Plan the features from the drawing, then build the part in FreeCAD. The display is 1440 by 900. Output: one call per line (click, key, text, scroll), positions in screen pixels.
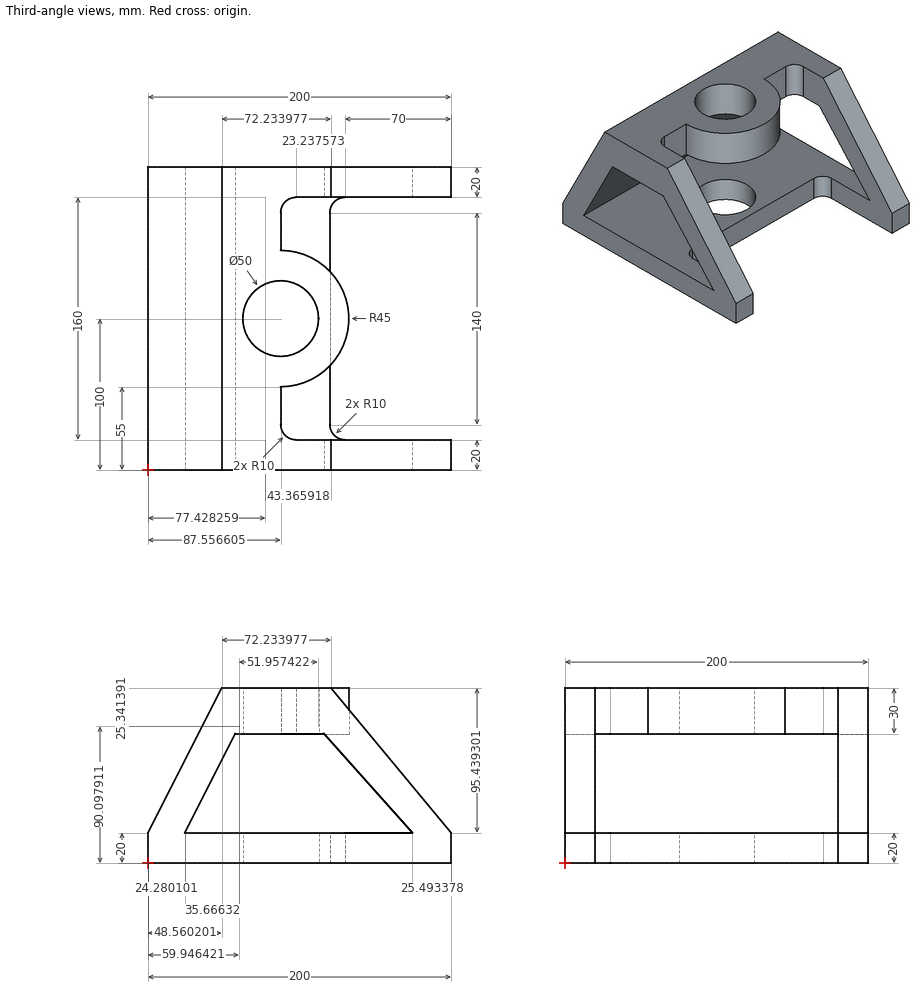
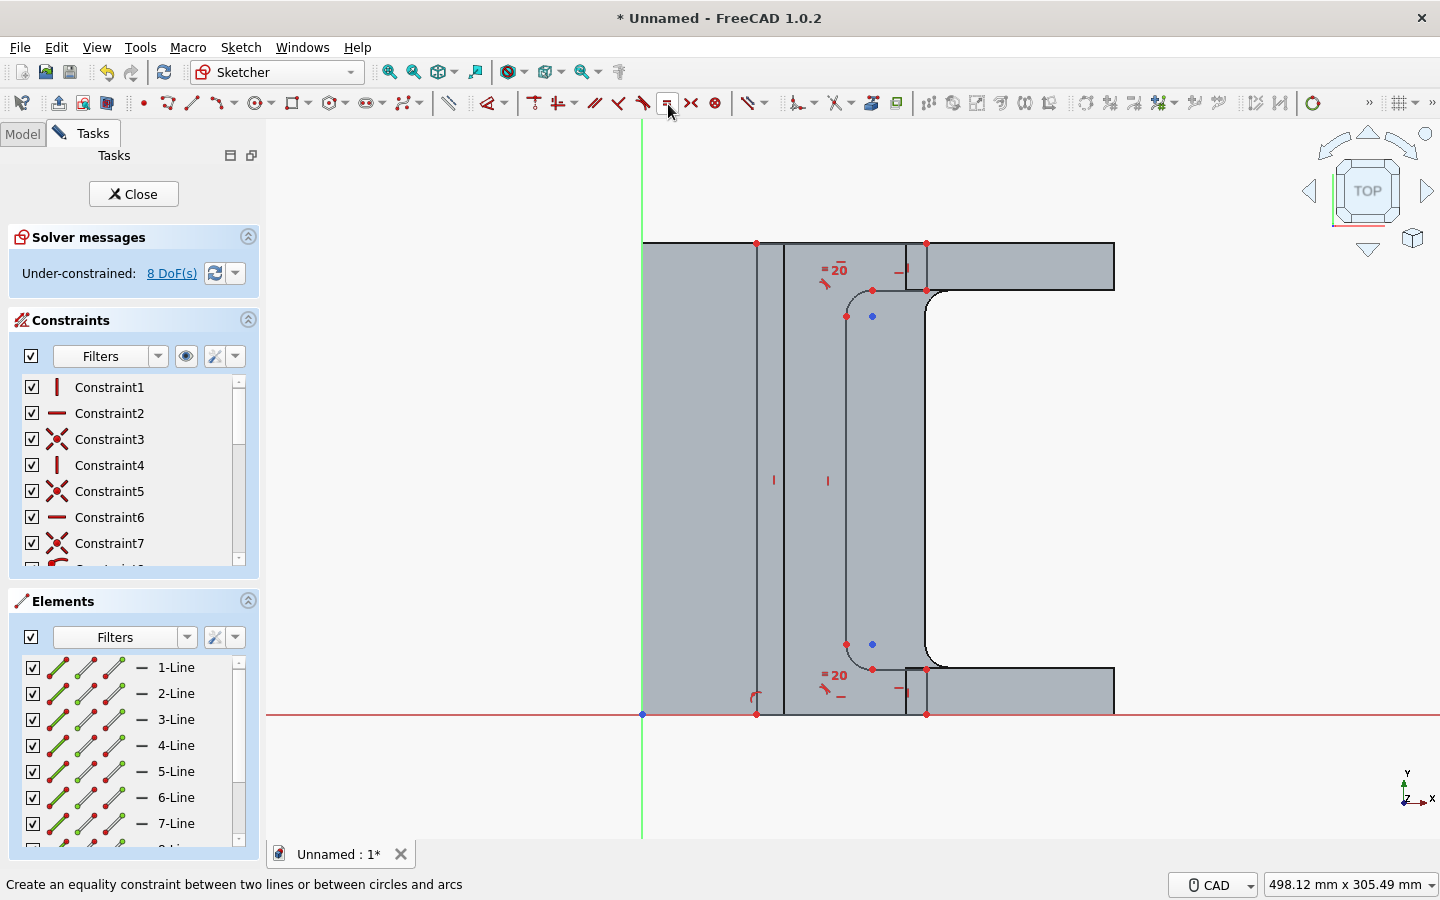
click(488, 104)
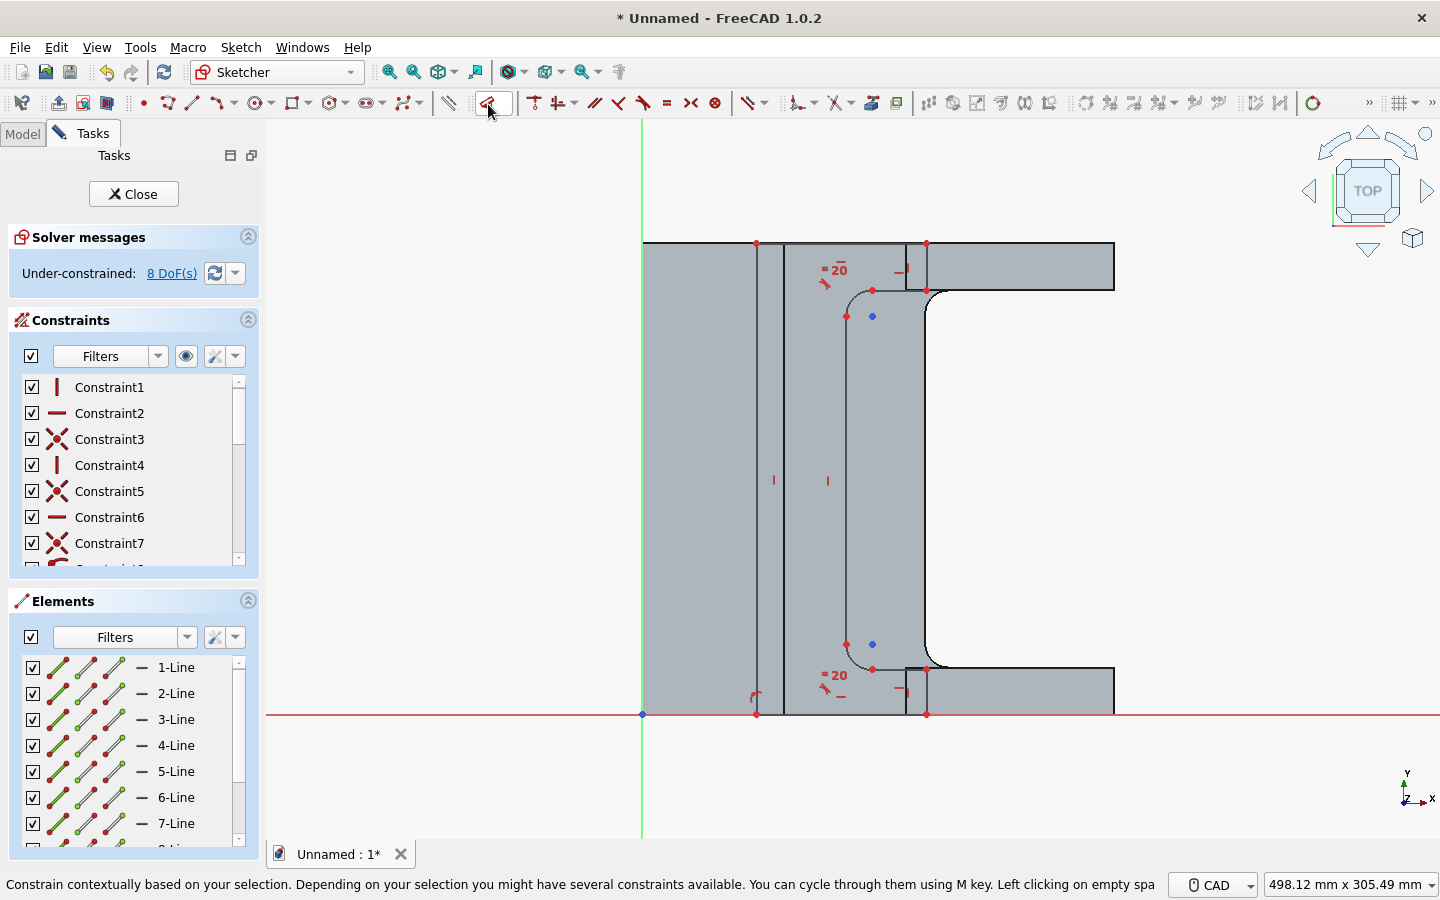
scroll(860, 293, up, 3)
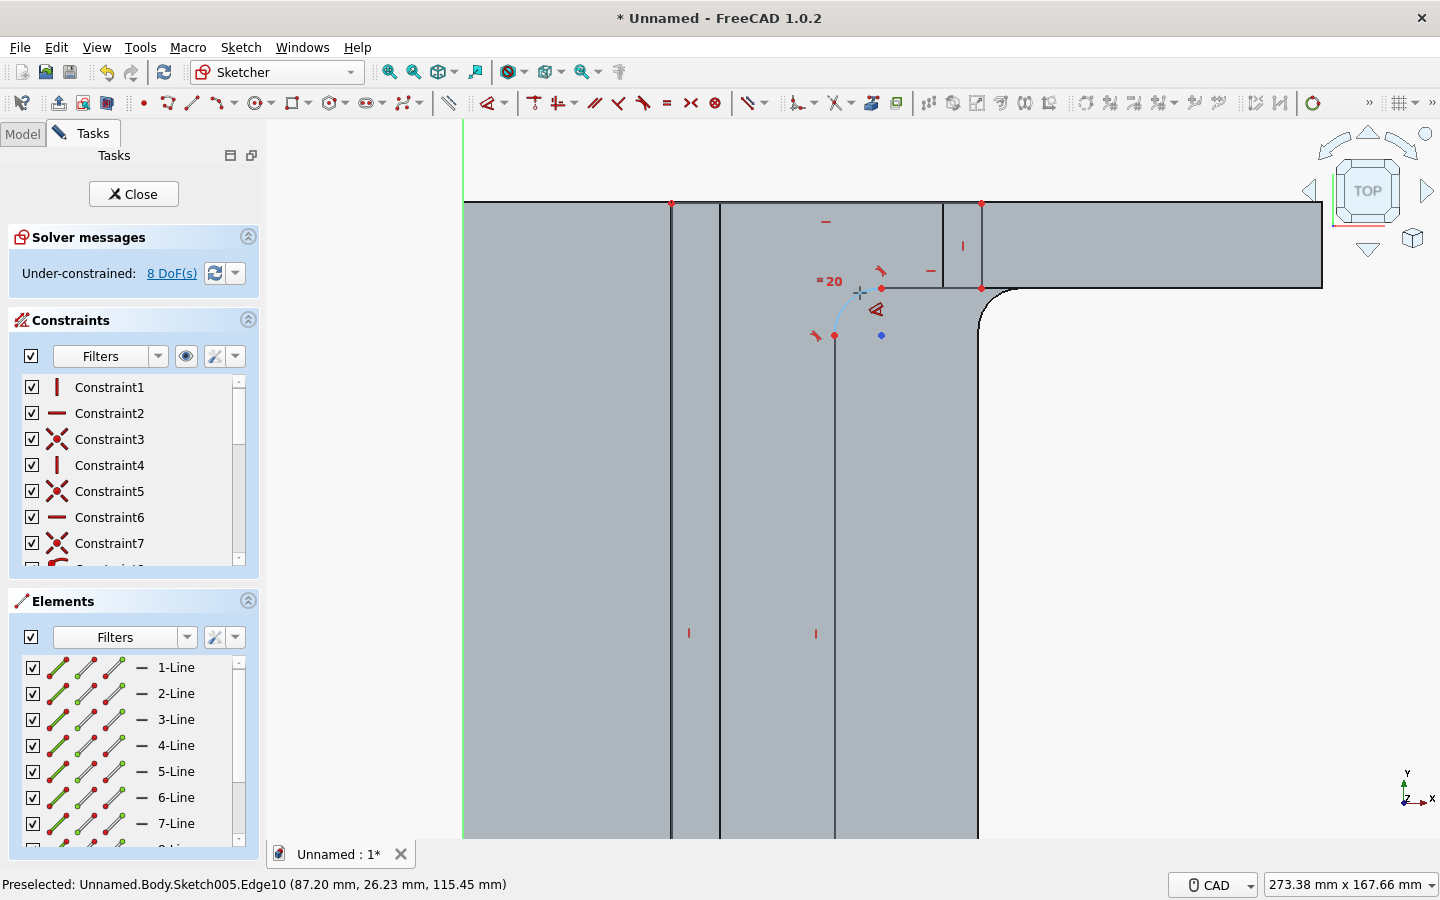
click(860, 293)
click(845, 265)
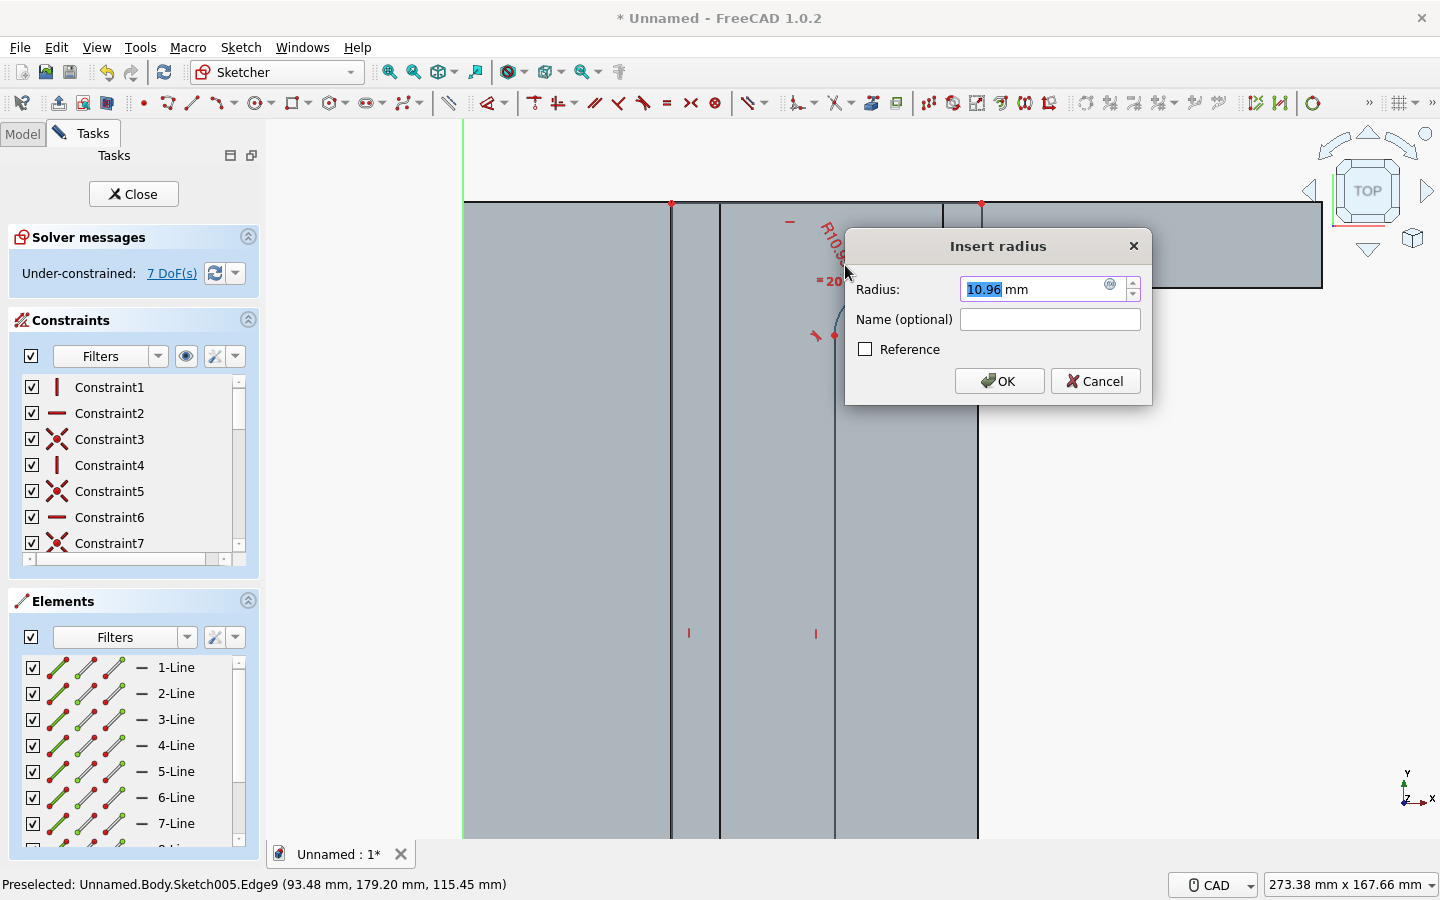
text(10)
key(Return)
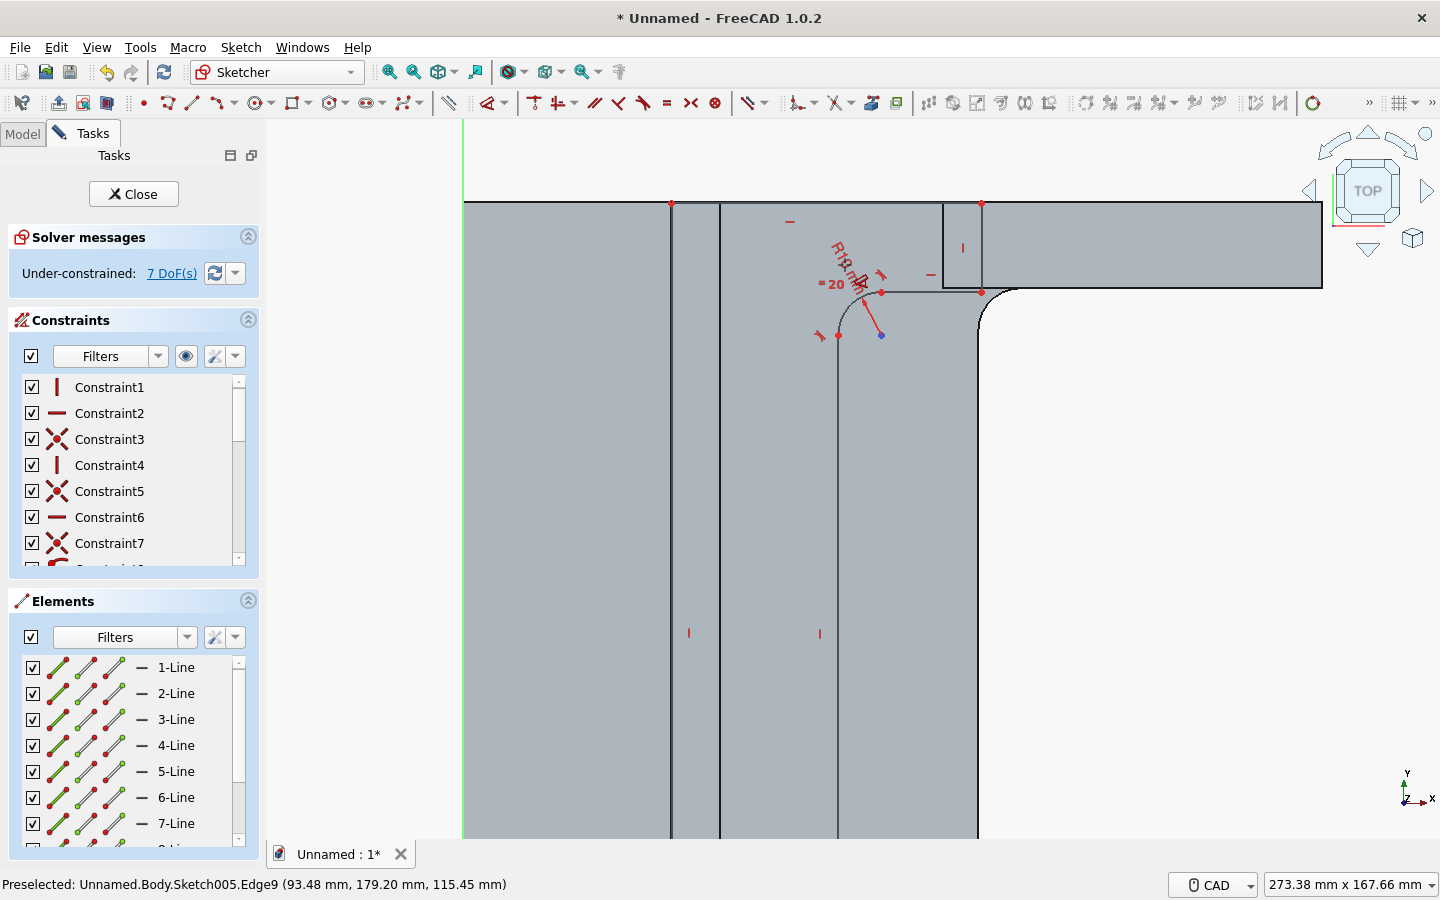
click(982, 266)
click(1016, 248)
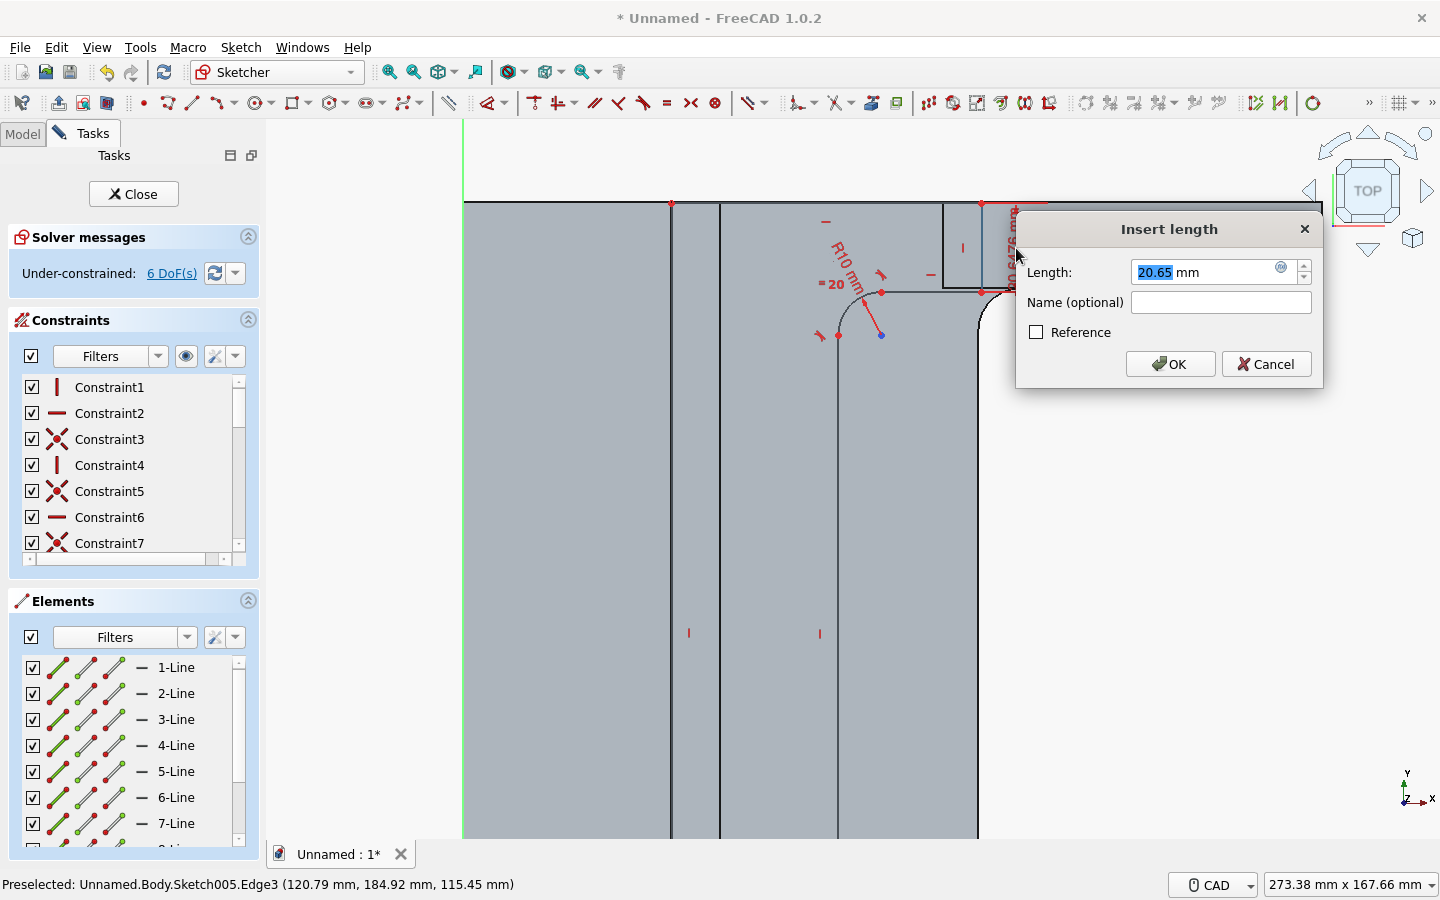
text(20)
key(Return)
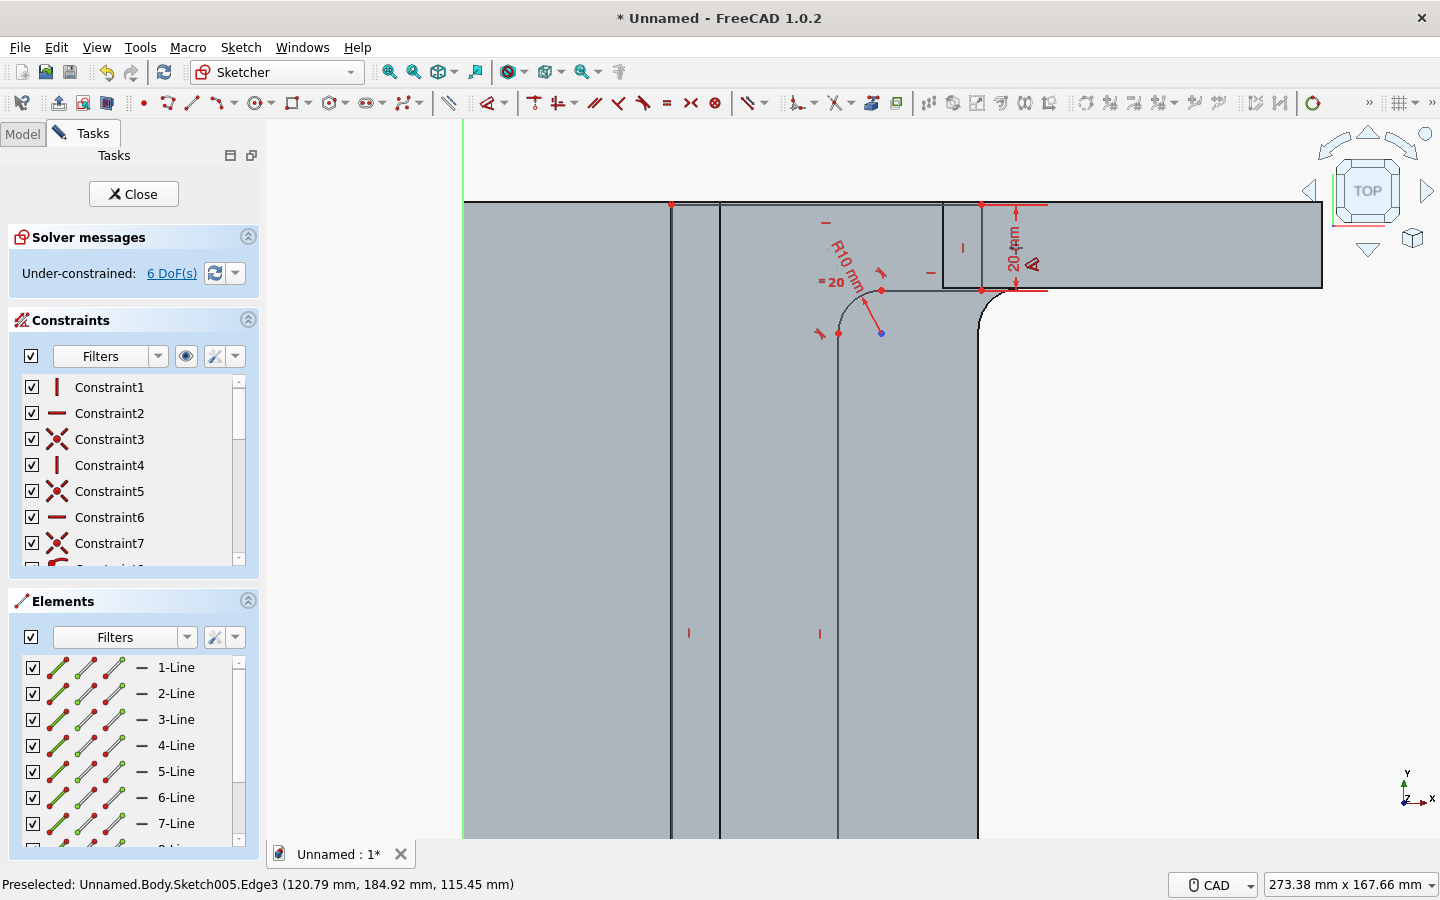
scroll(860, 293, down, 3)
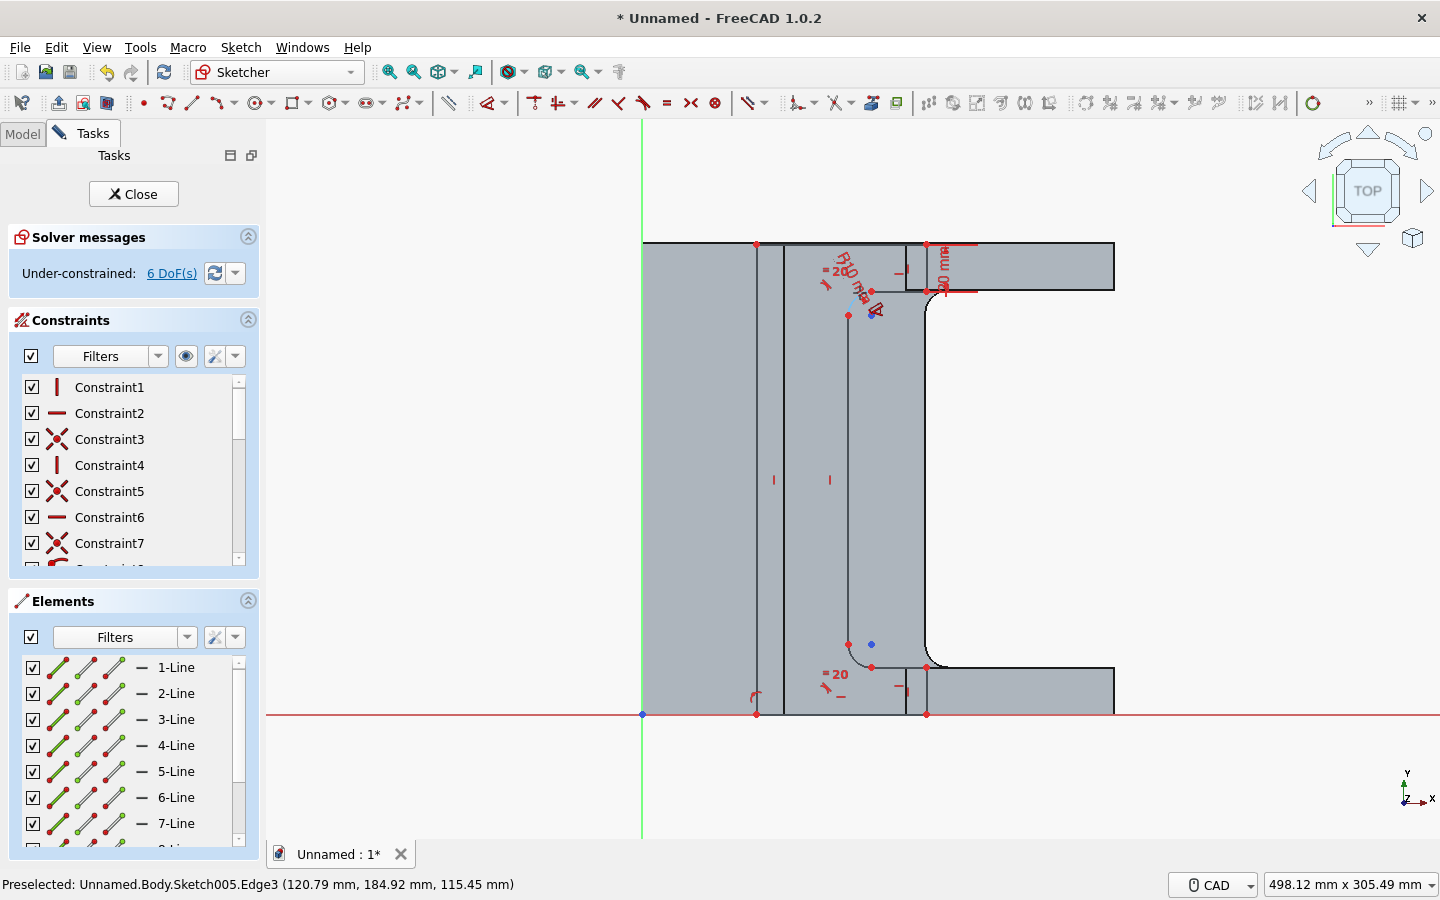
click(927, 701)
click(961, 691)